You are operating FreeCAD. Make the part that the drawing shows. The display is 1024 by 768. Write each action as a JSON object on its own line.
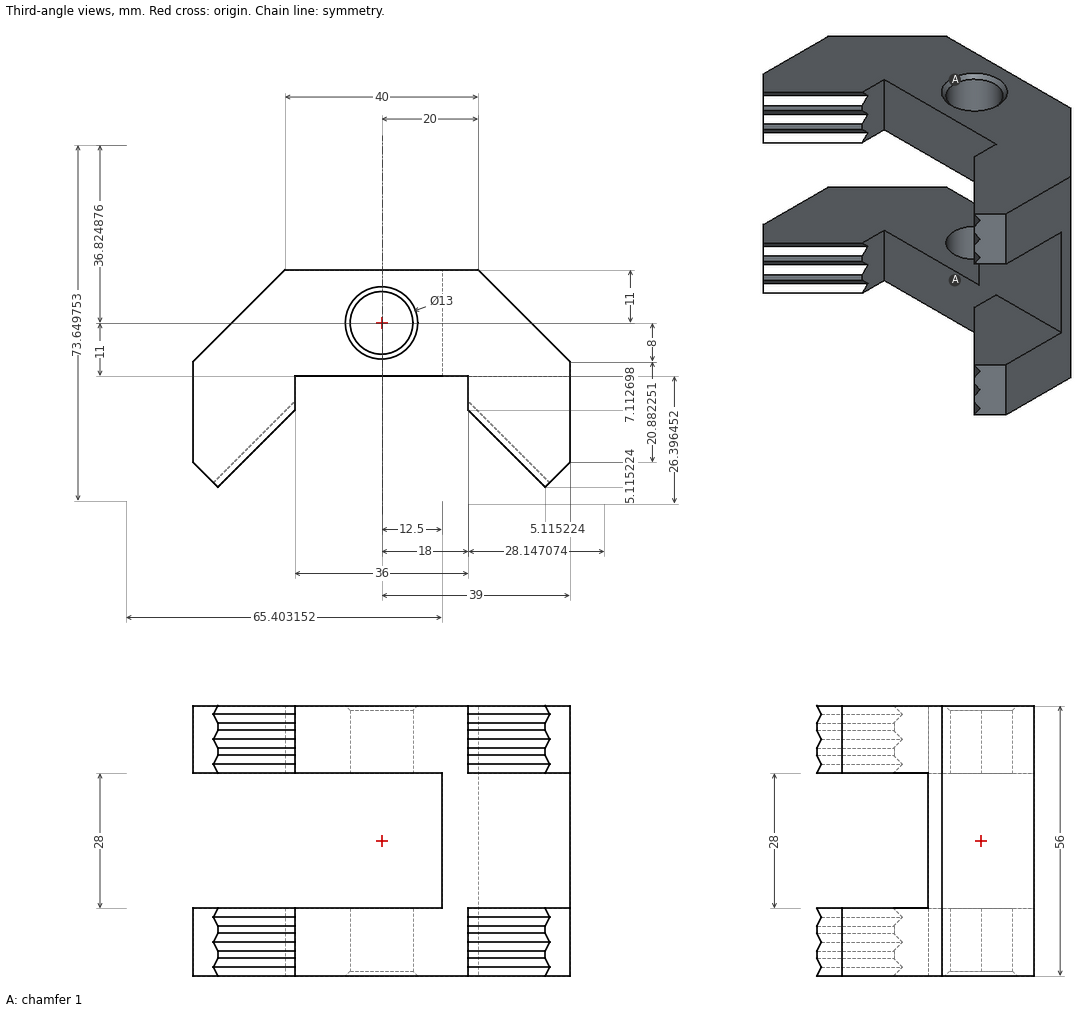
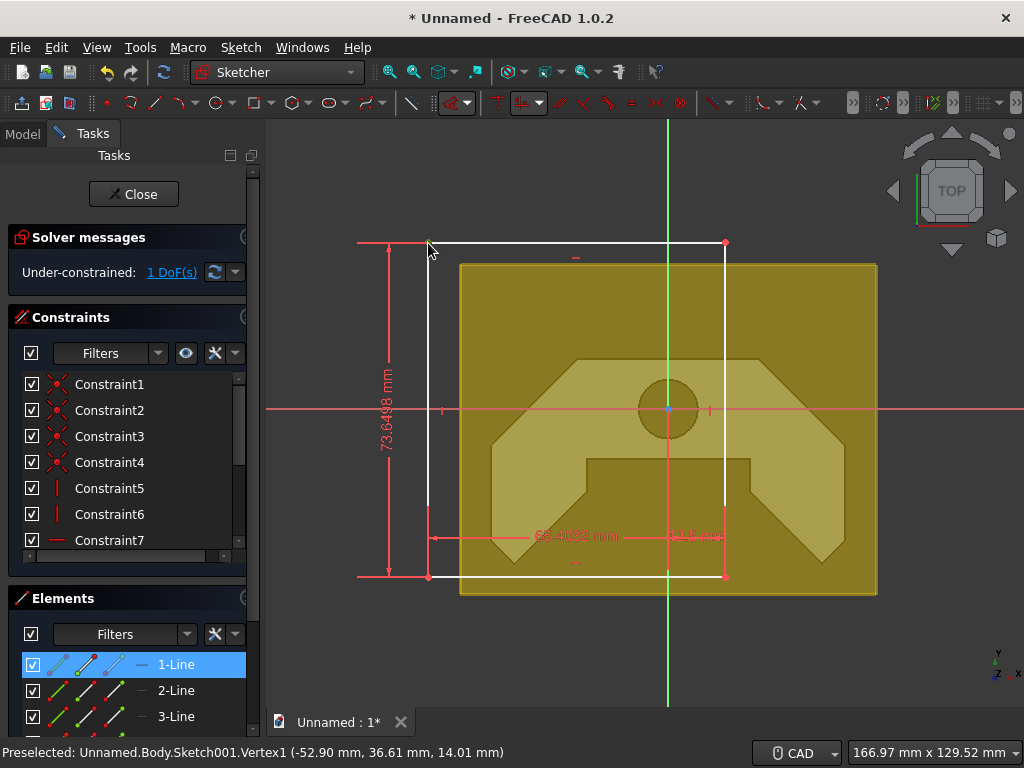
{"action": "left_click", "coordinate": [470, 104]}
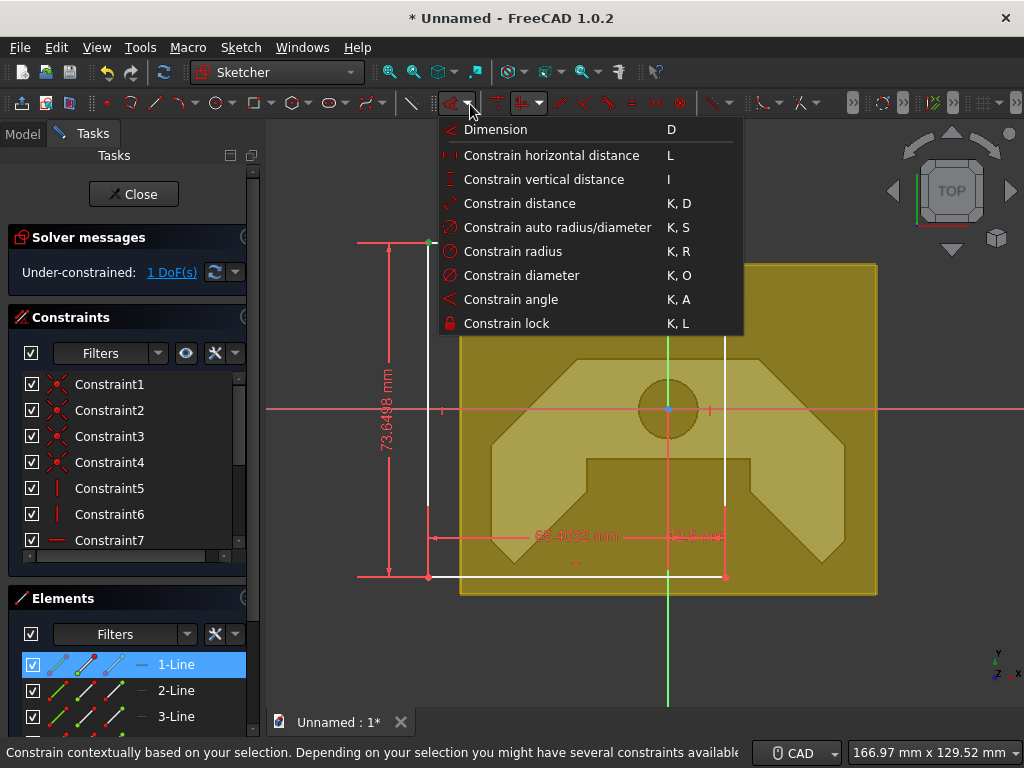
{"action": "left_click", "coordinate": [591, 179]}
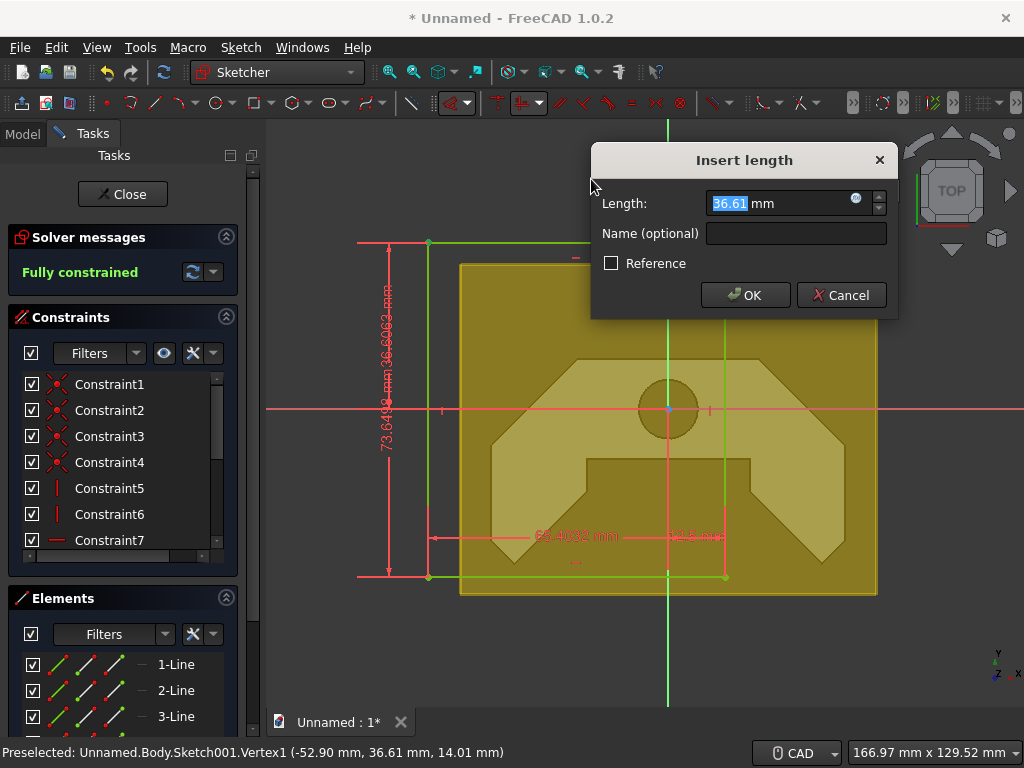
{"action": "type", "text": "36.824876"}
{"action": "key", "text": "Return"}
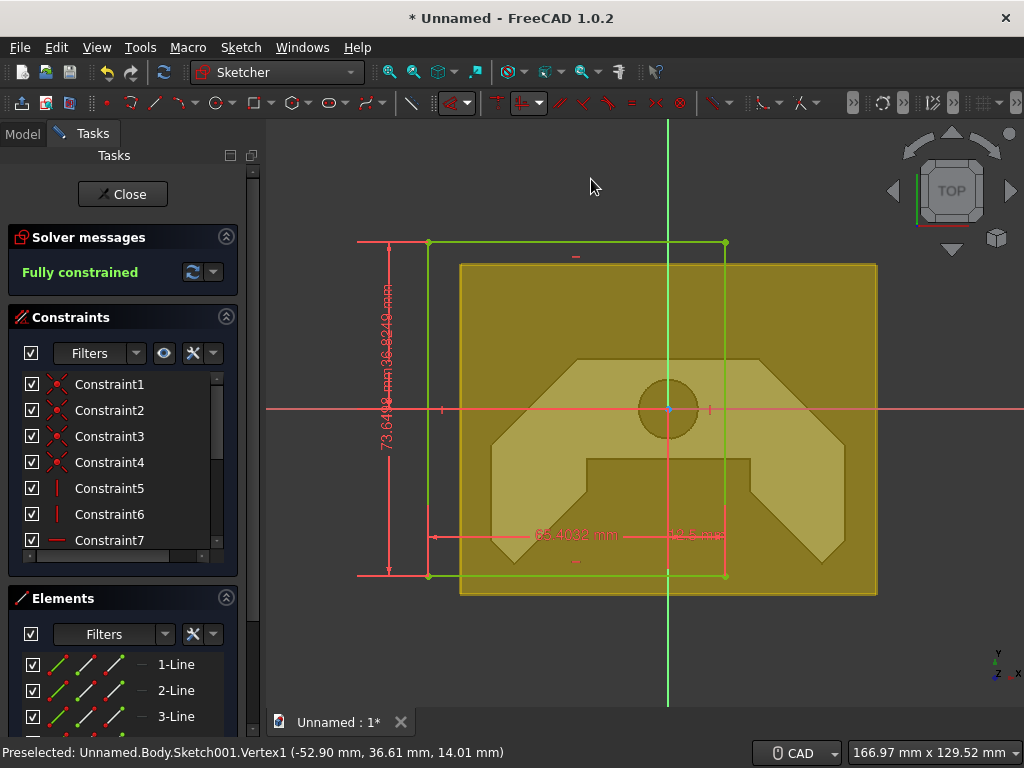
{"action": "left_click", "coordinate": [123, 194]}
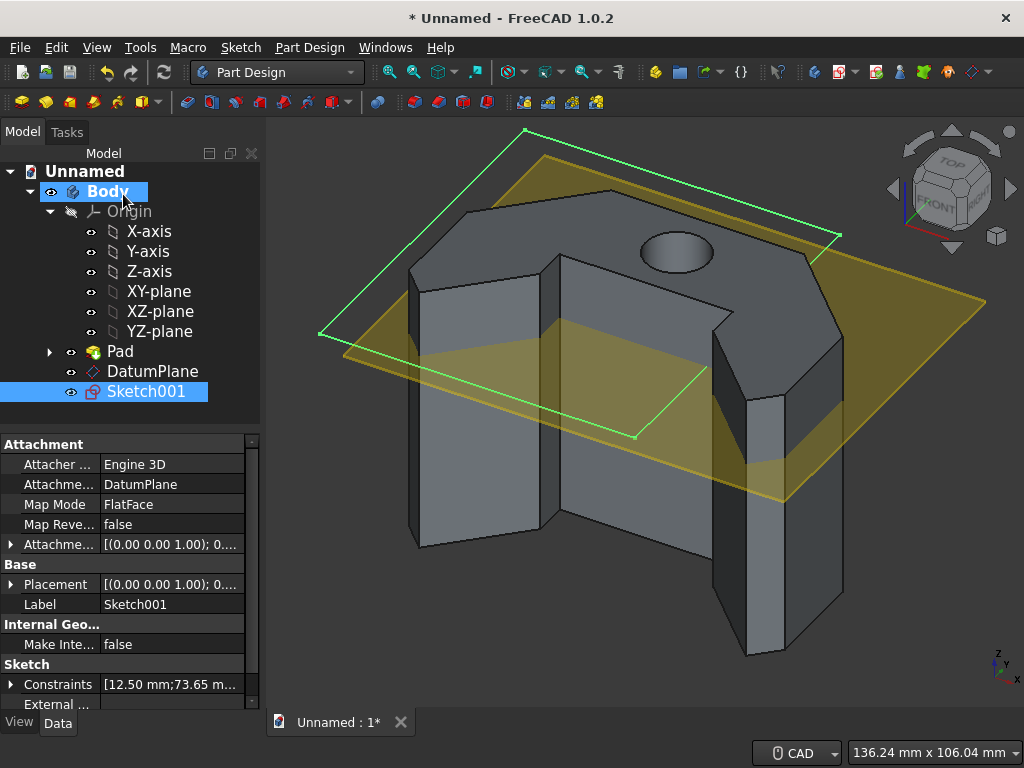
{"action": "left_click", "coordinate": [188, 102]}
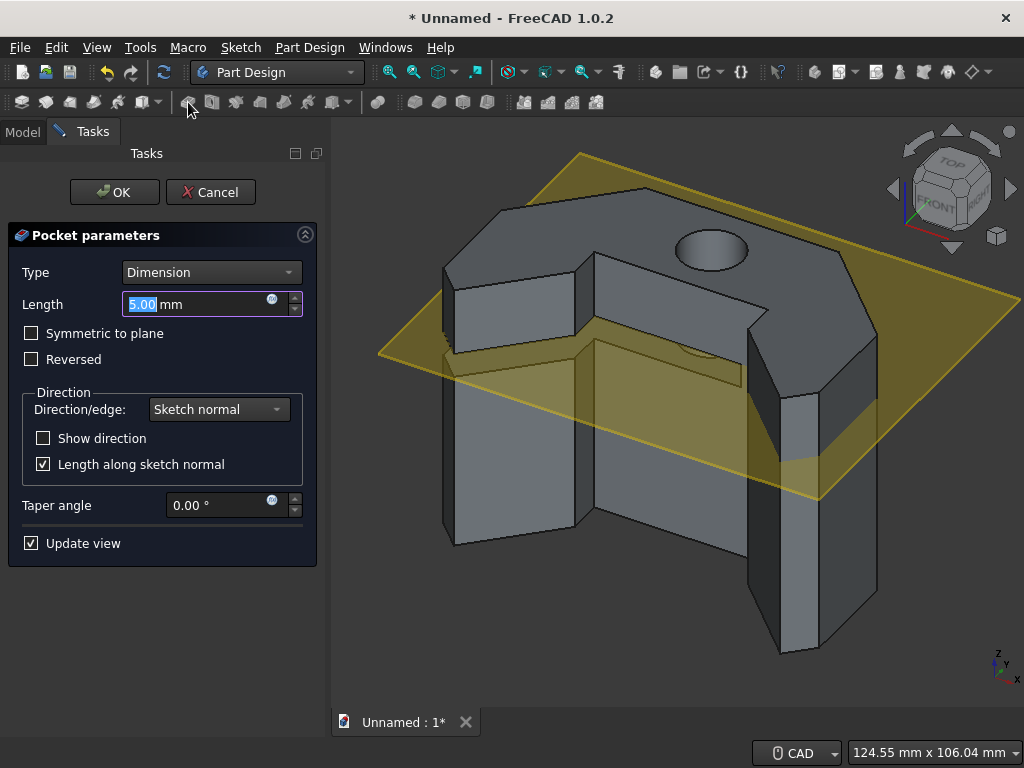
{"action": "type", "text": "28"}
{"action": "key", "text": "Tab"}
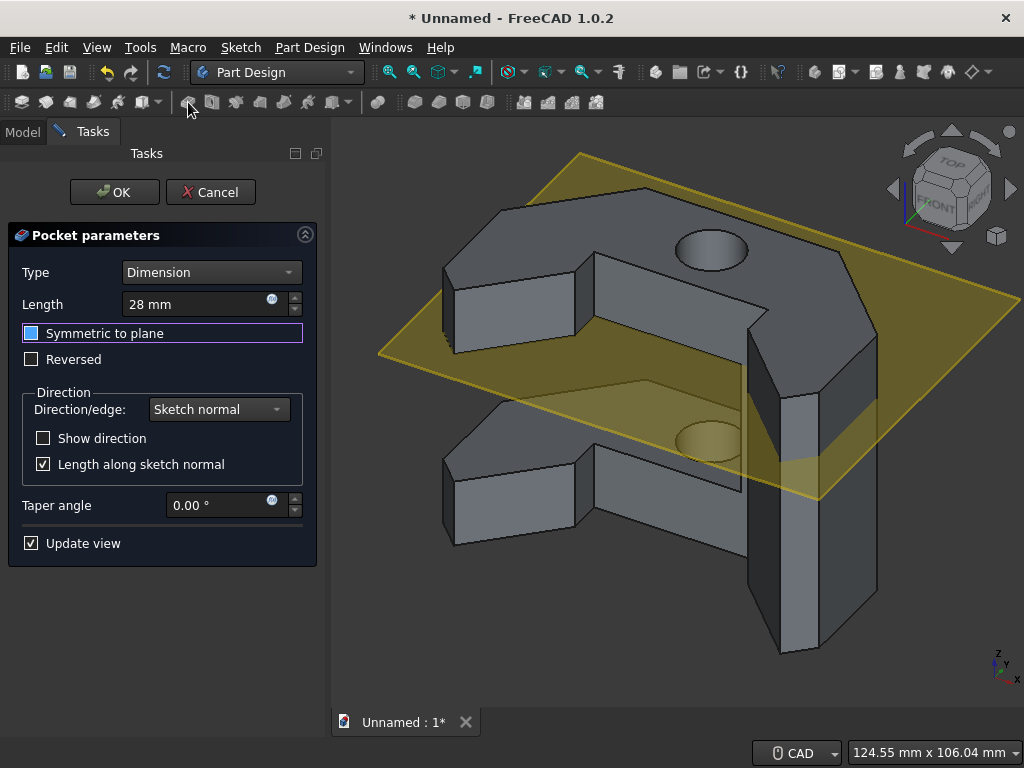
{"action": "left_click", "coordinate": [115, 192]}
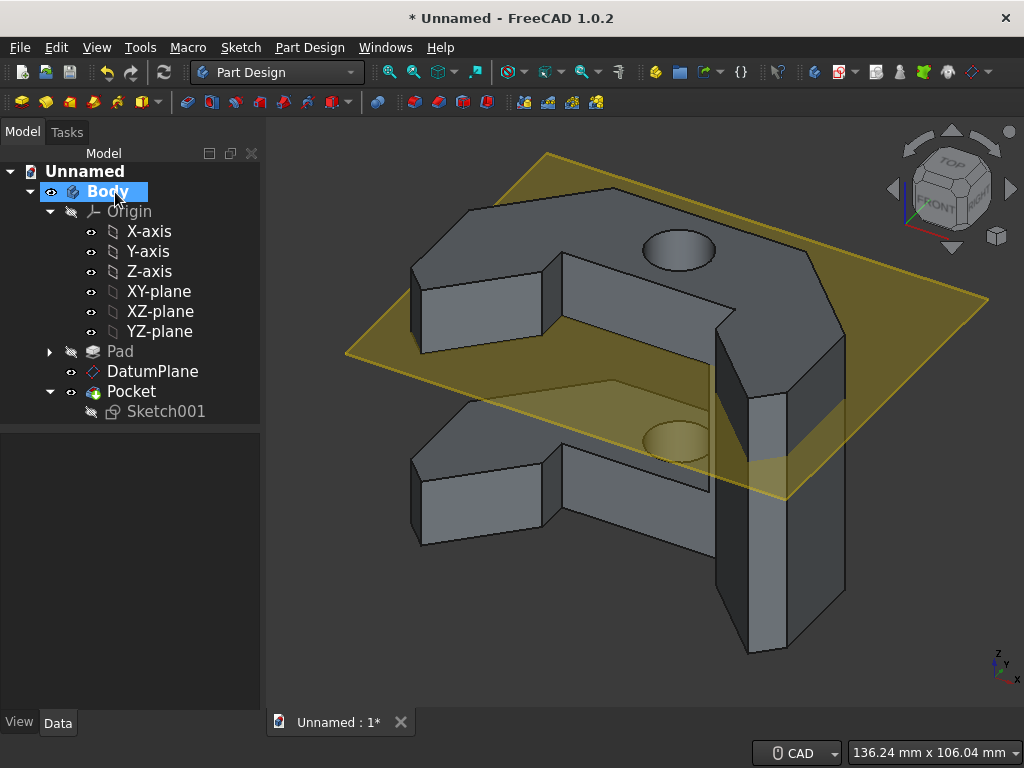
{"action": "left_click", "coordinate": [116, 372]}
{"action": "key", "text": "space"}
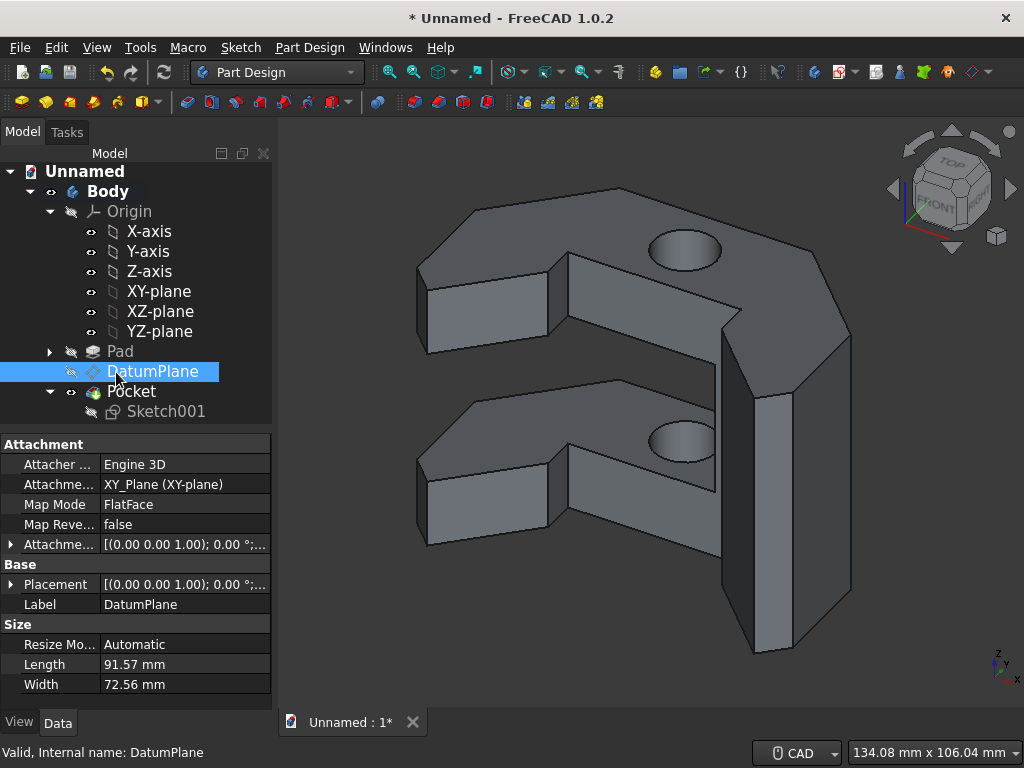
{"action": "key", "text": "6"}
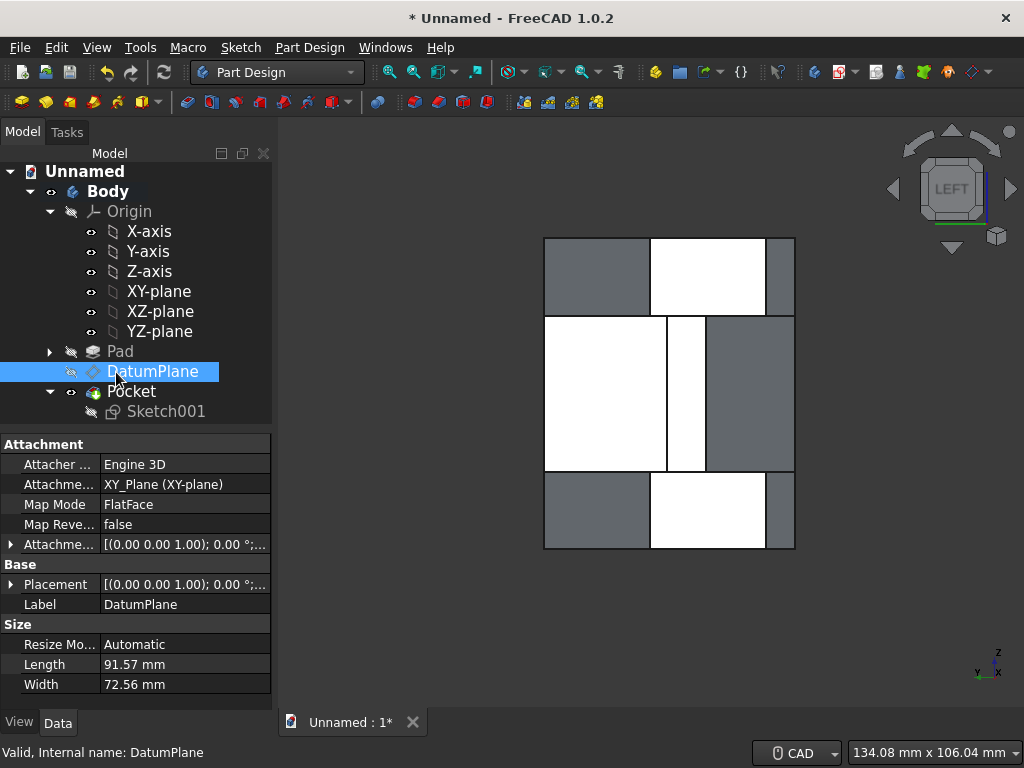
{"action": "left_click", "coordinate": [780, 265]}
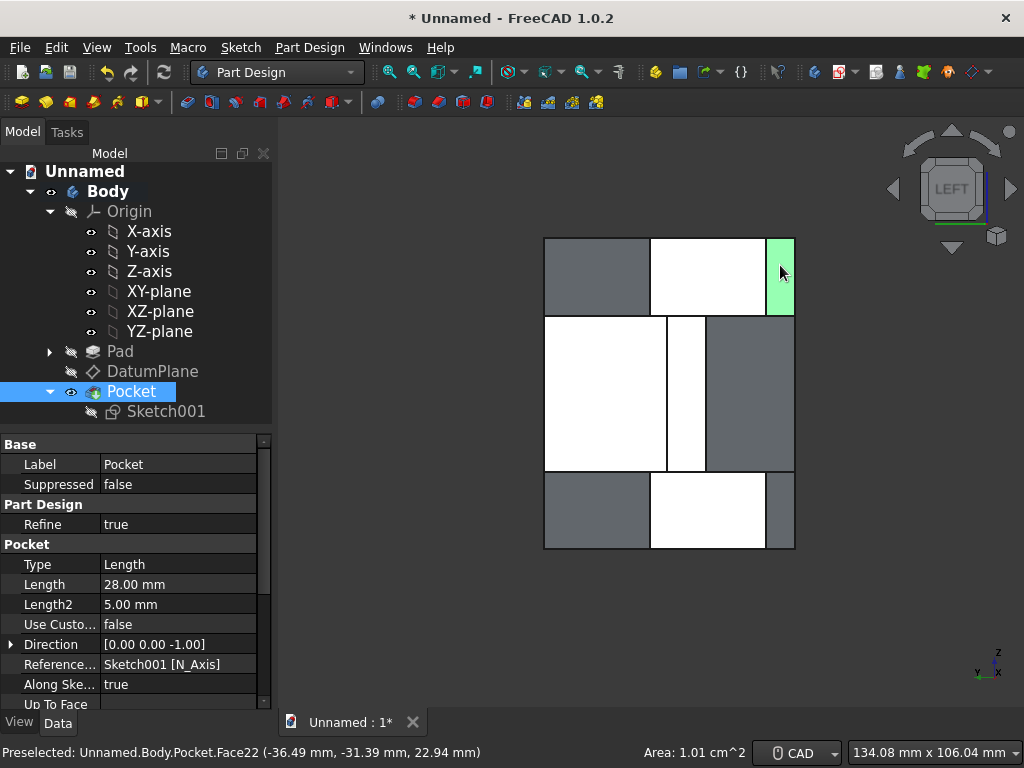
{"action": "left_click", "coordinate": [840, 72]}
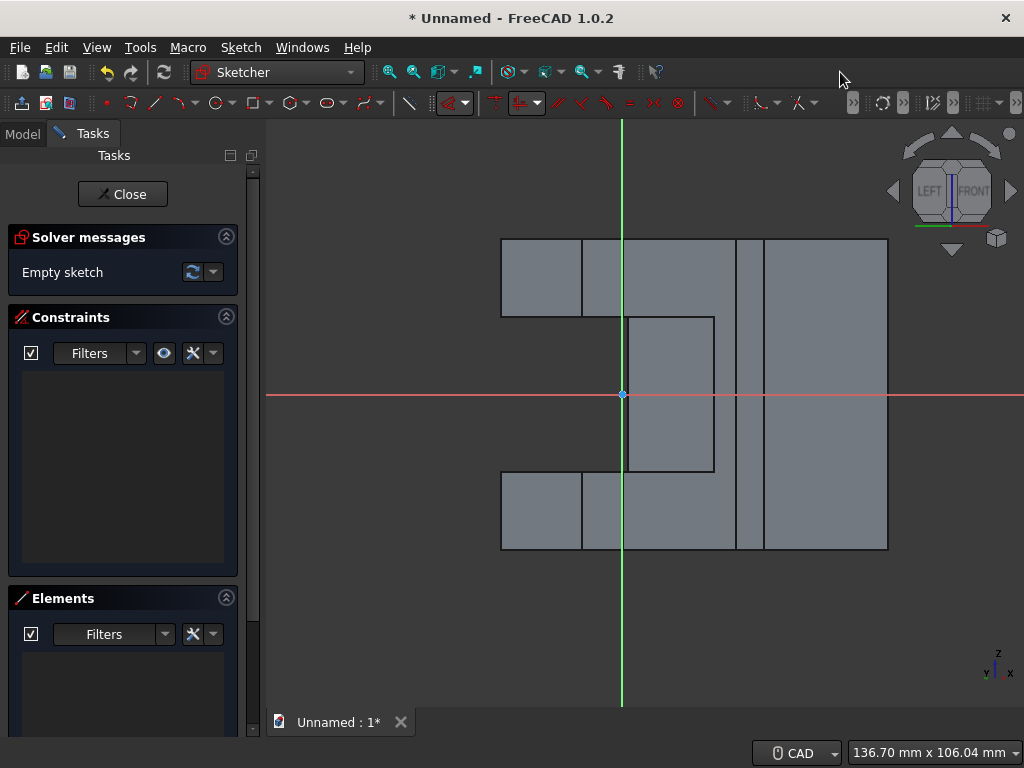
{"action": "key", "text": "q s"}